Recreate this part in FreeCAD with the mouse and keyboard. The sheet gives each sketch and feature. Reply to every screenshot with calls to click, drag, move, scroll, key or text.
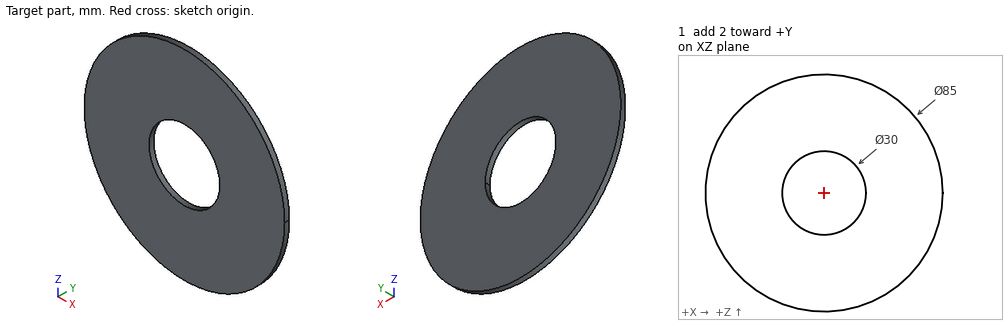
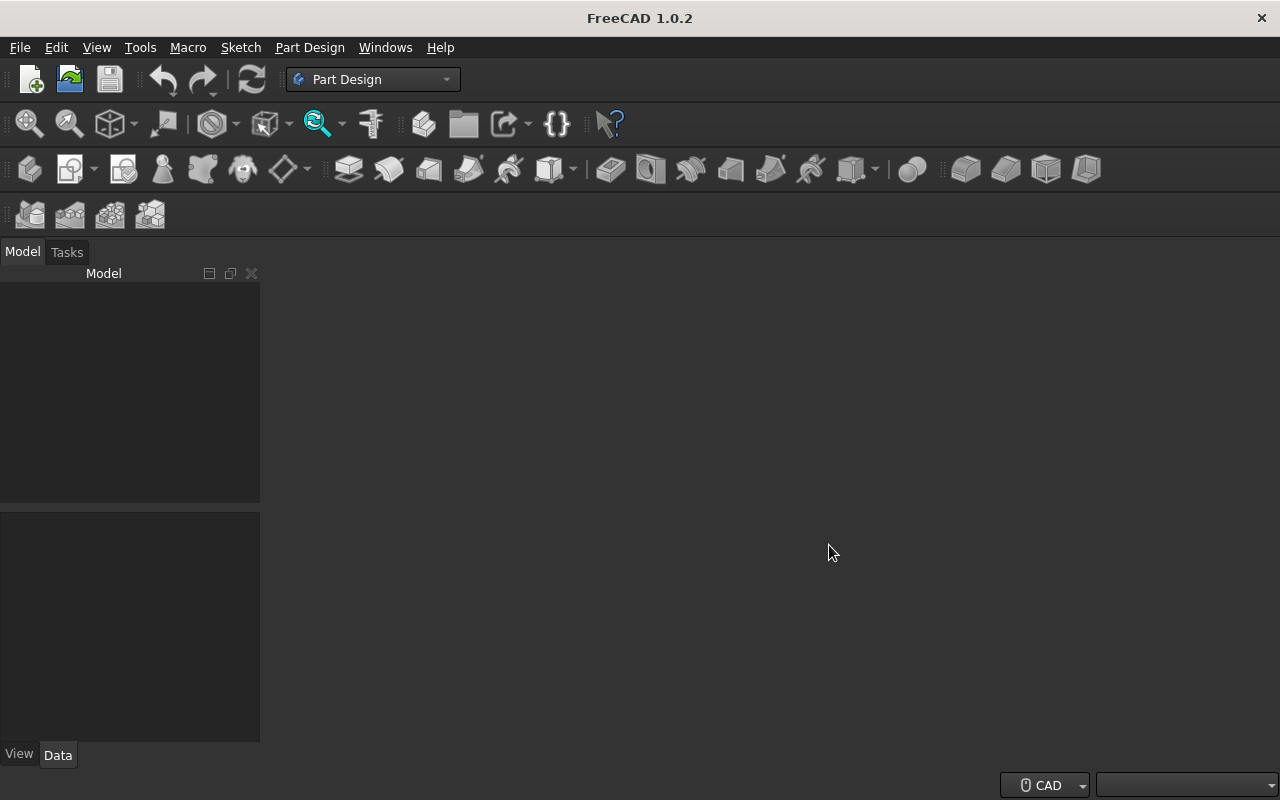
click(30, 80)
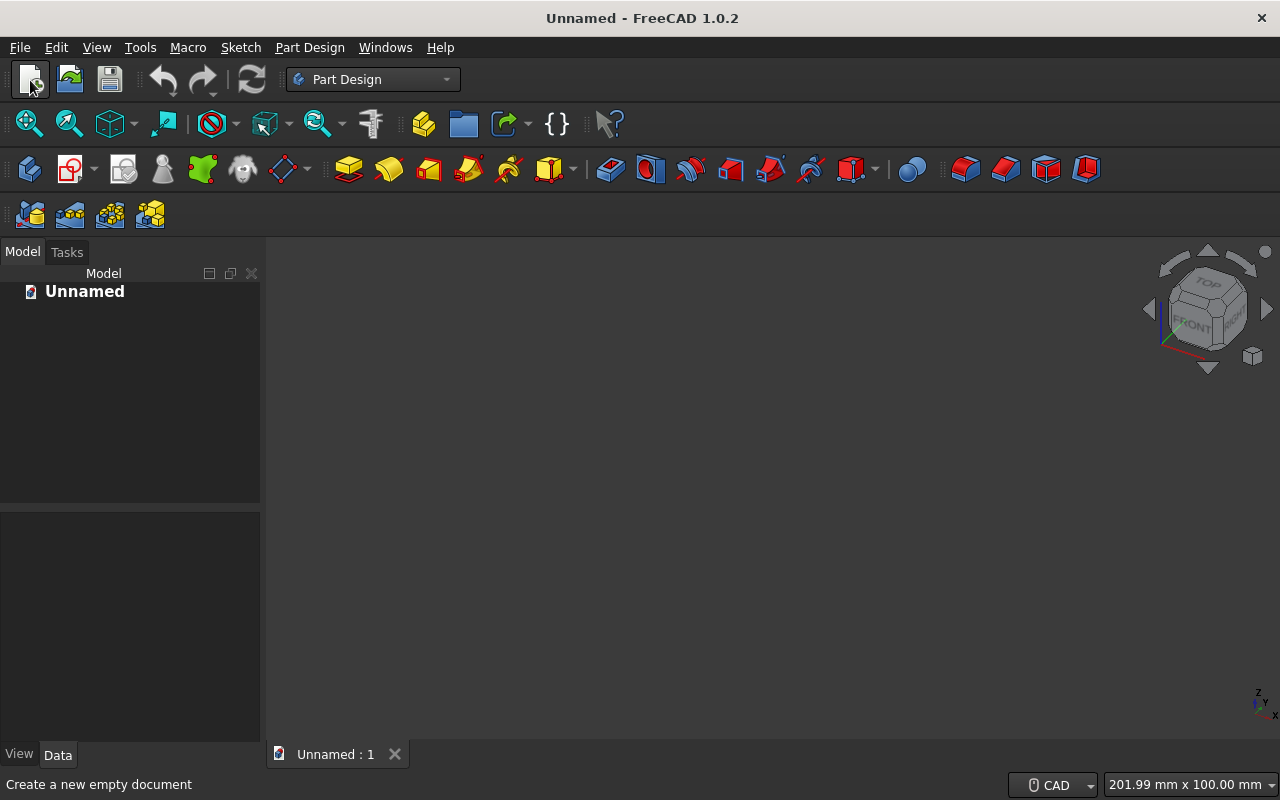
click(70, 170)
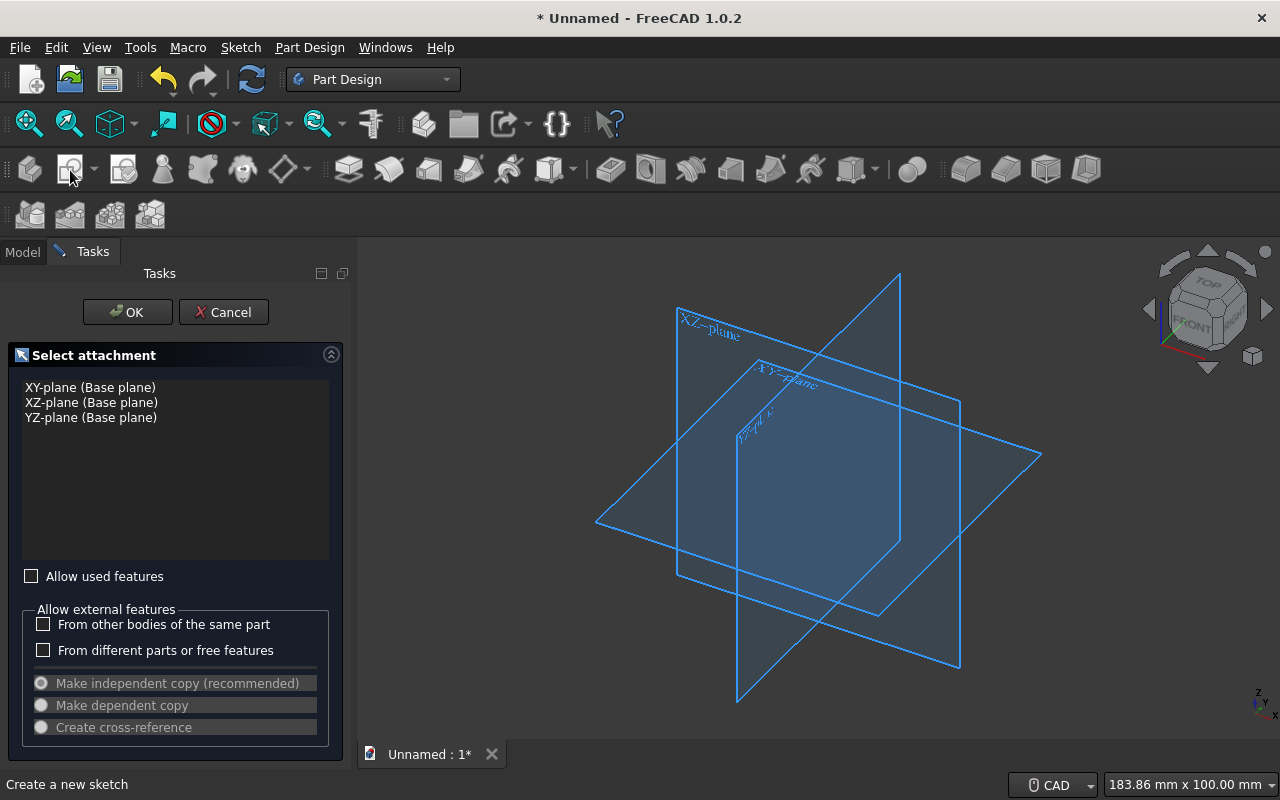
click(82, 402)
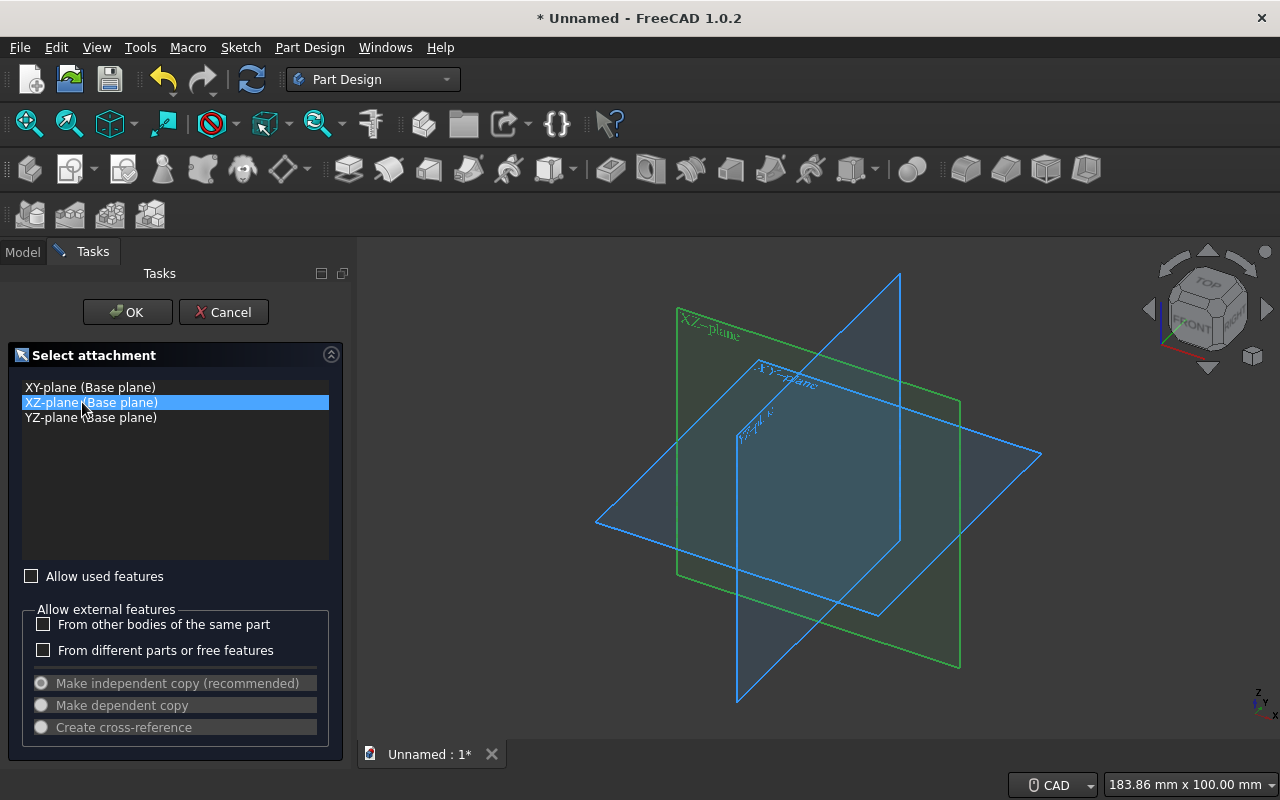
click(128, 312)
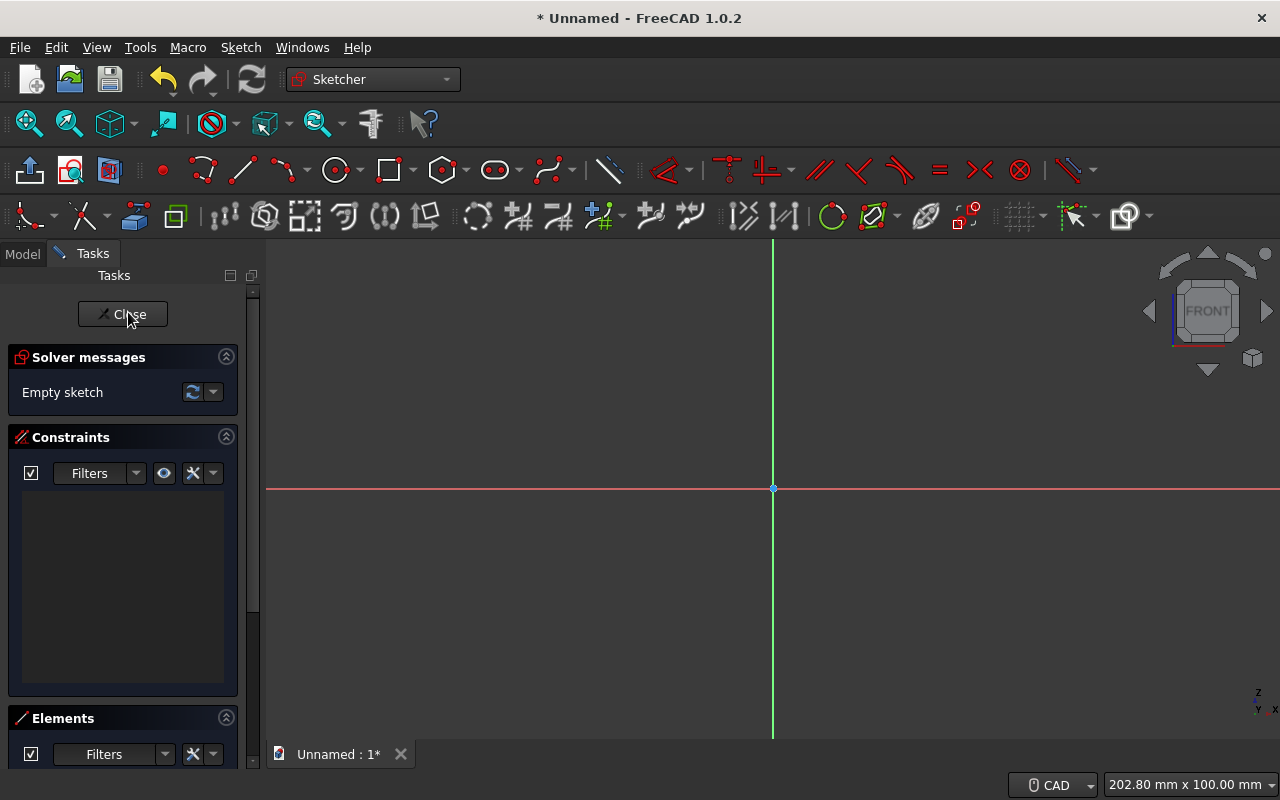
scroll(565, 489, down, 2)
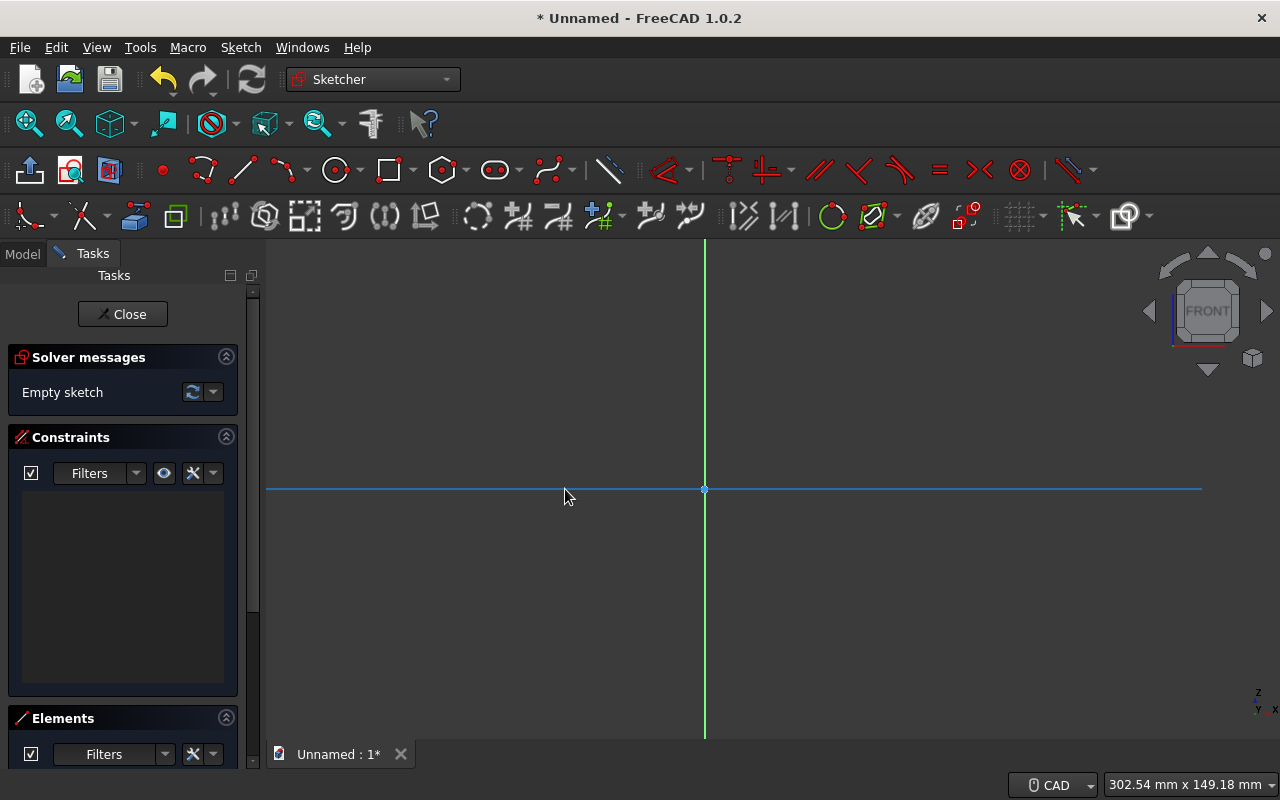
click(336, 170)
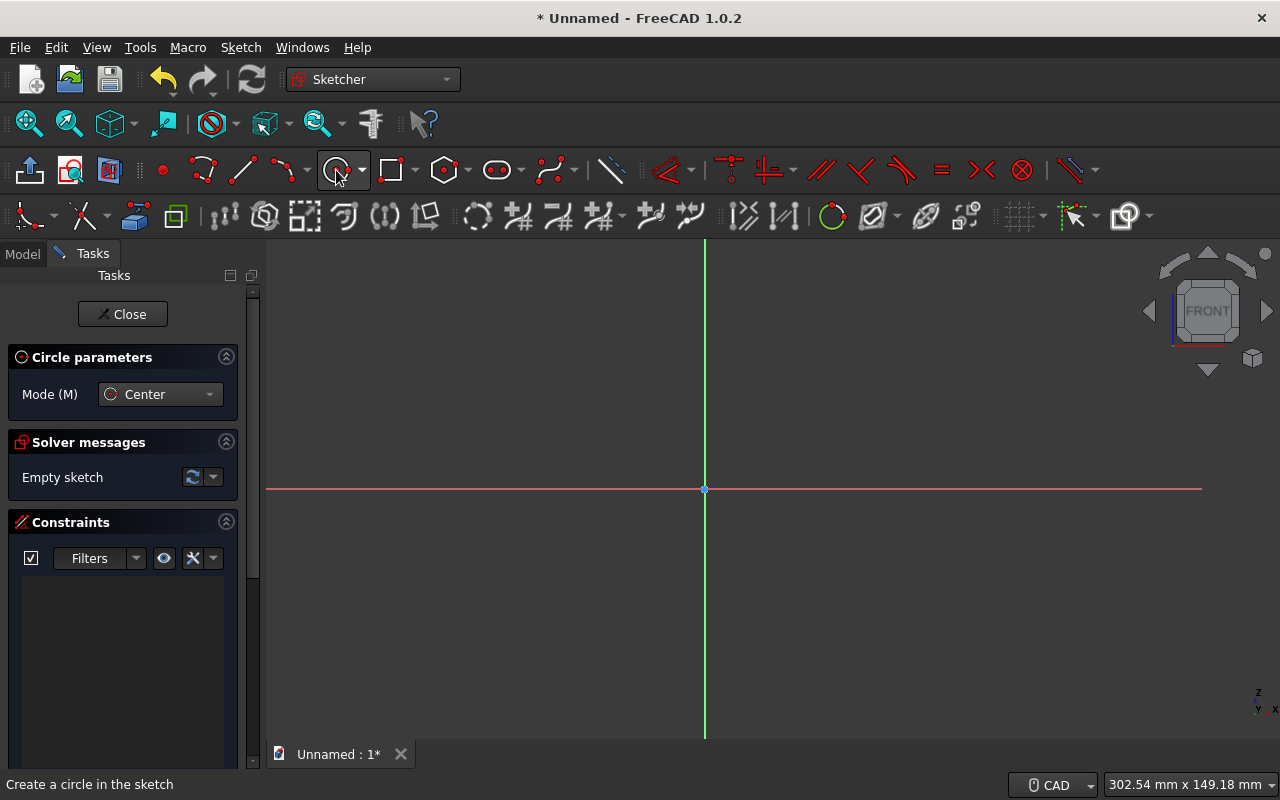
click(705, 489)
move(805, 388)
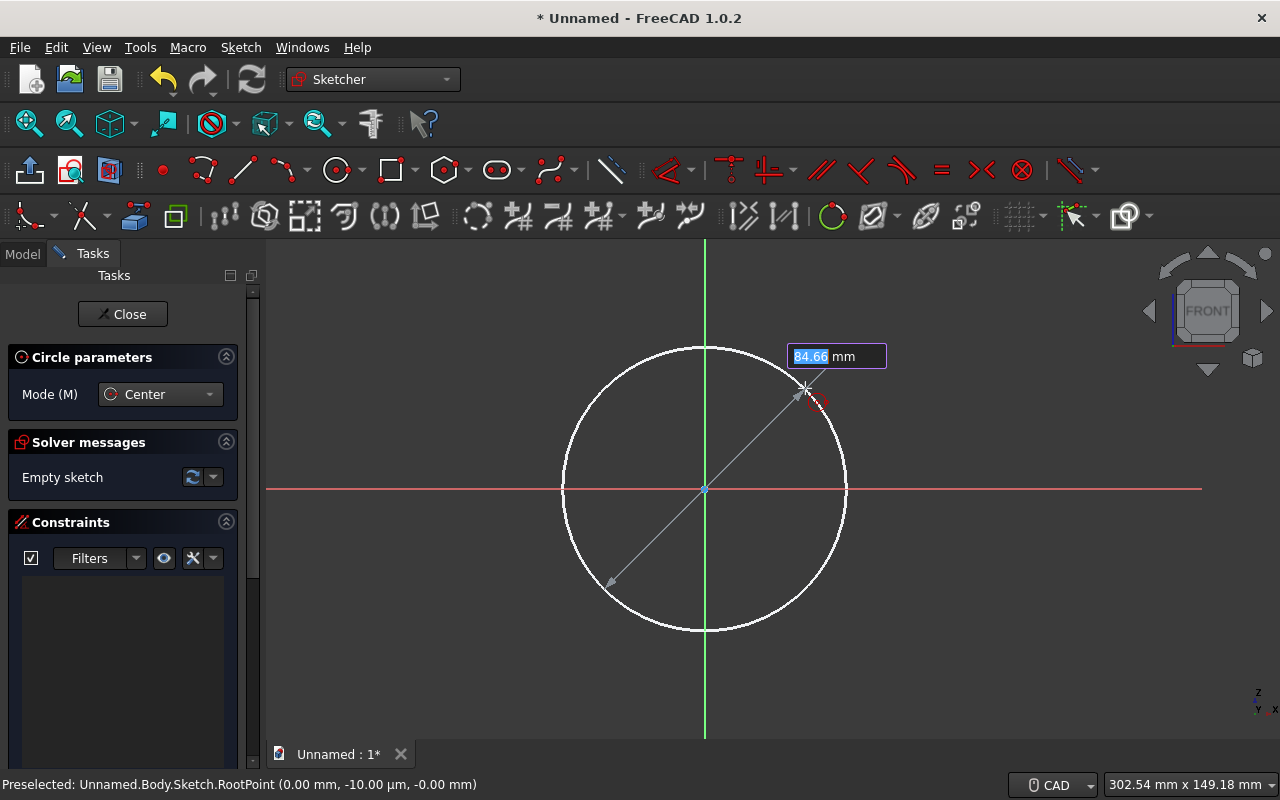
text(85)
key(Return)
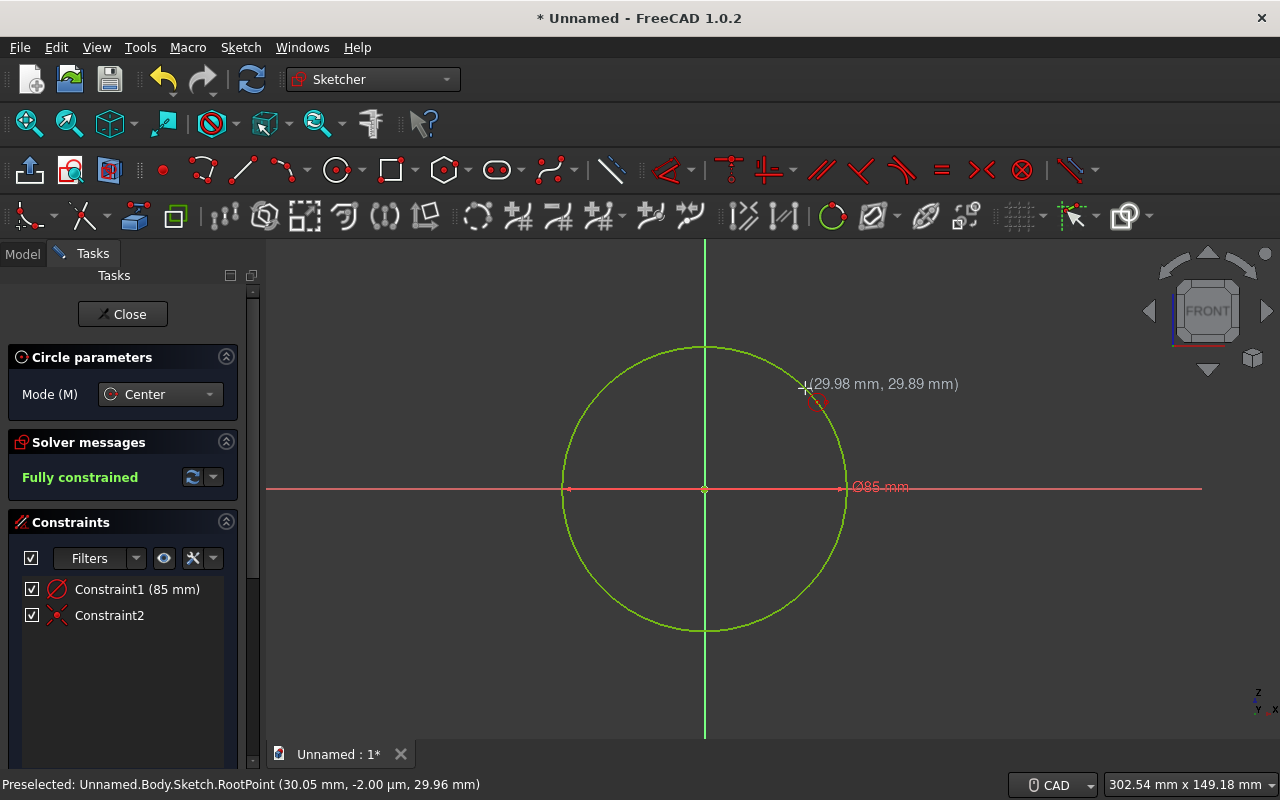
click(705, 489)
move(740, 454)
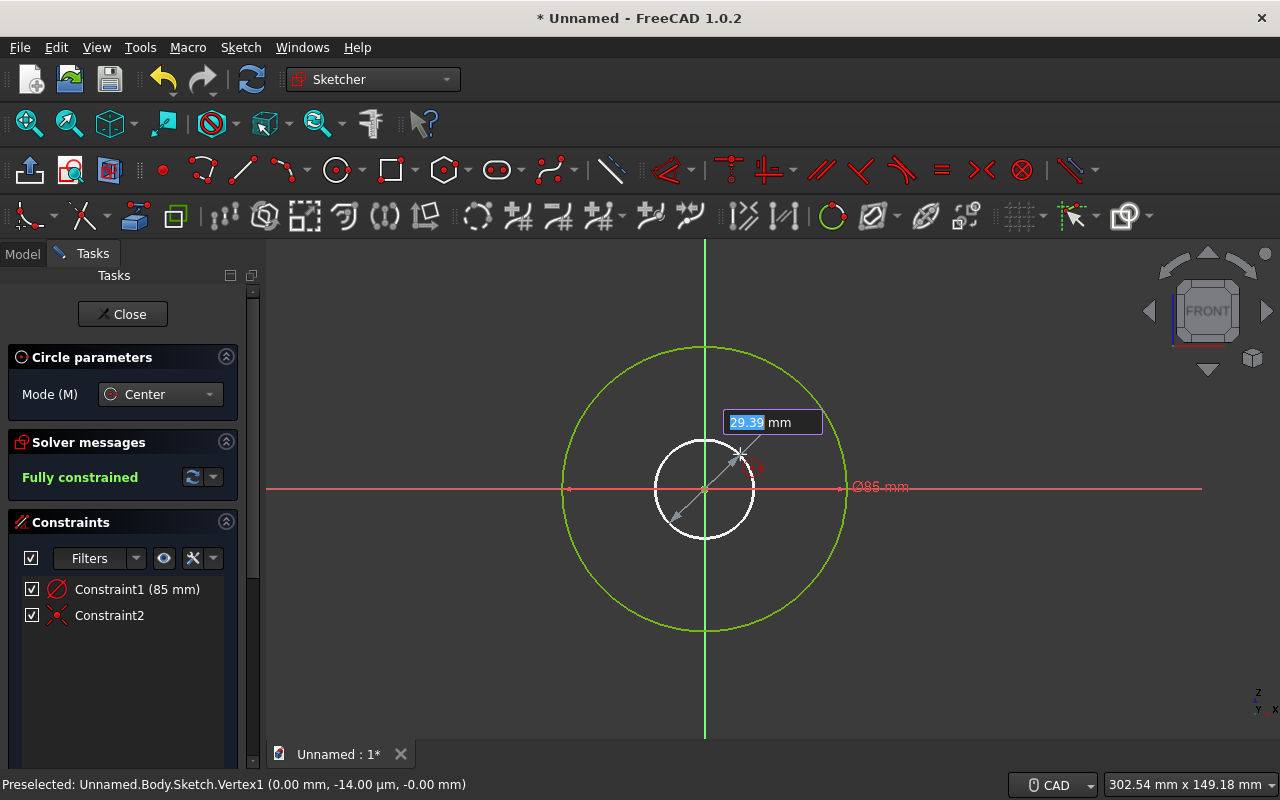
text(30)
key(Return)
key(Escape)